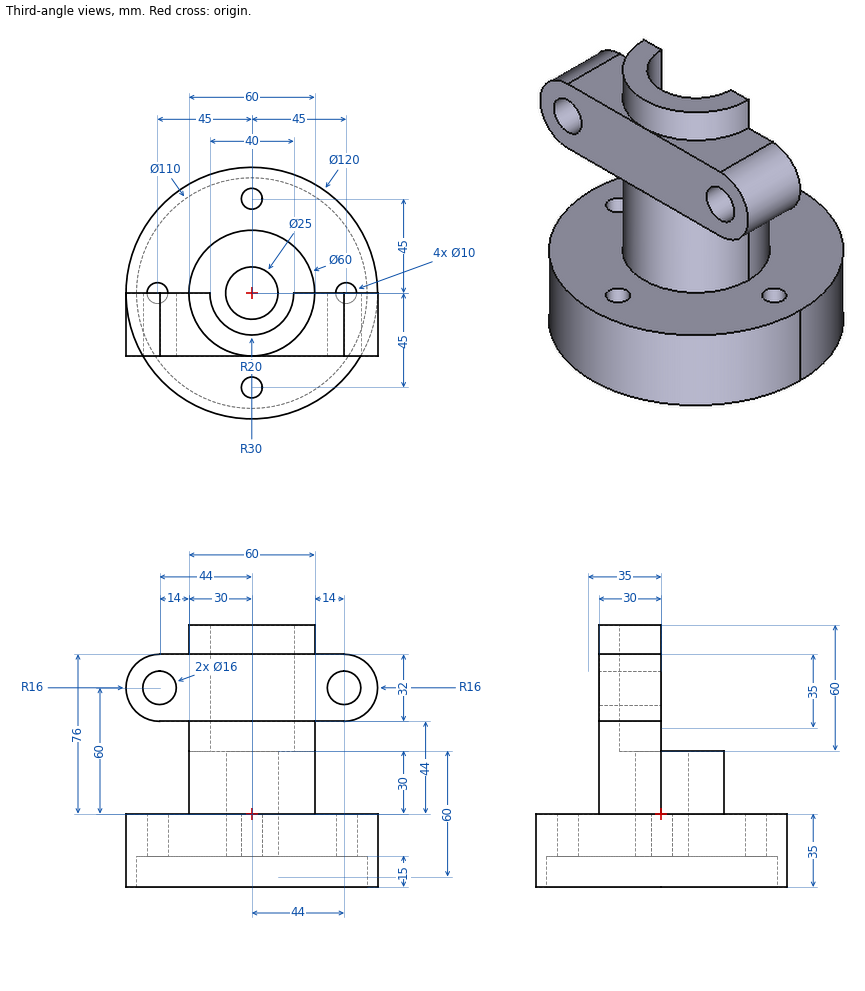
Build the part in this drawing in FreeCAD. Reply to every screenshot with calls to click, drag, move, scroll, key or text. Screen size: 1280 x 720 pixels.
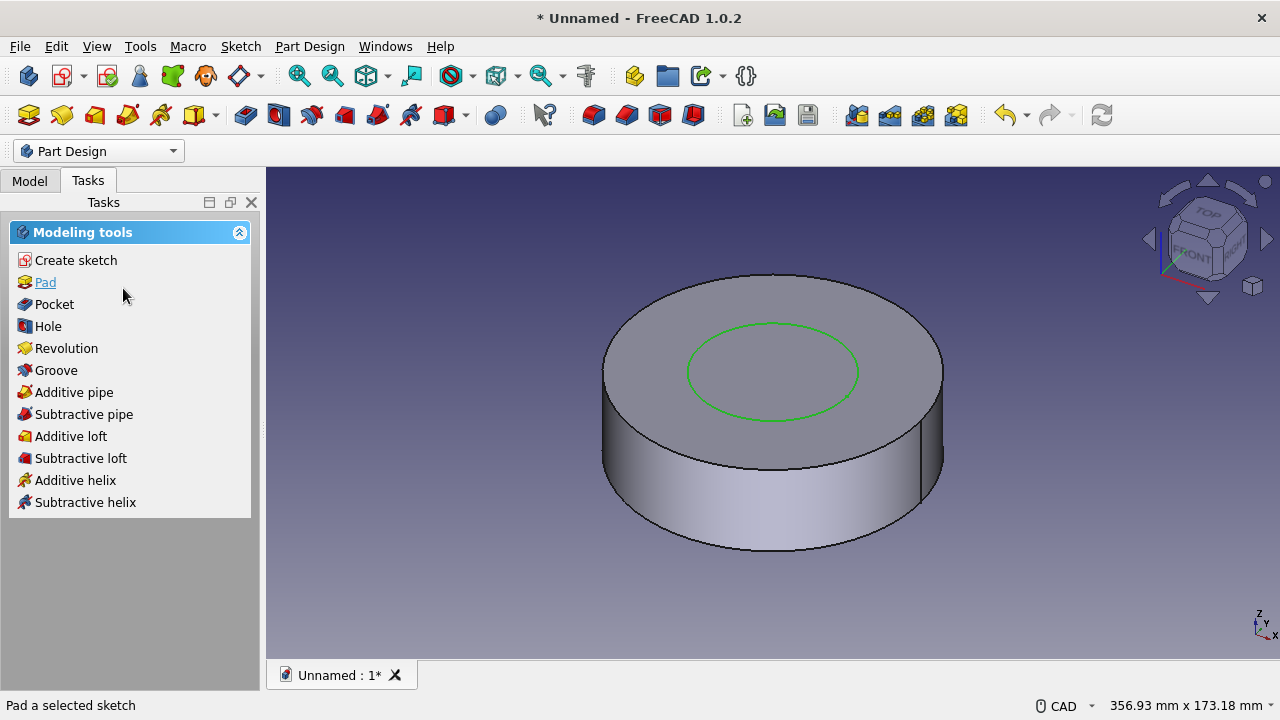
click(29, 116)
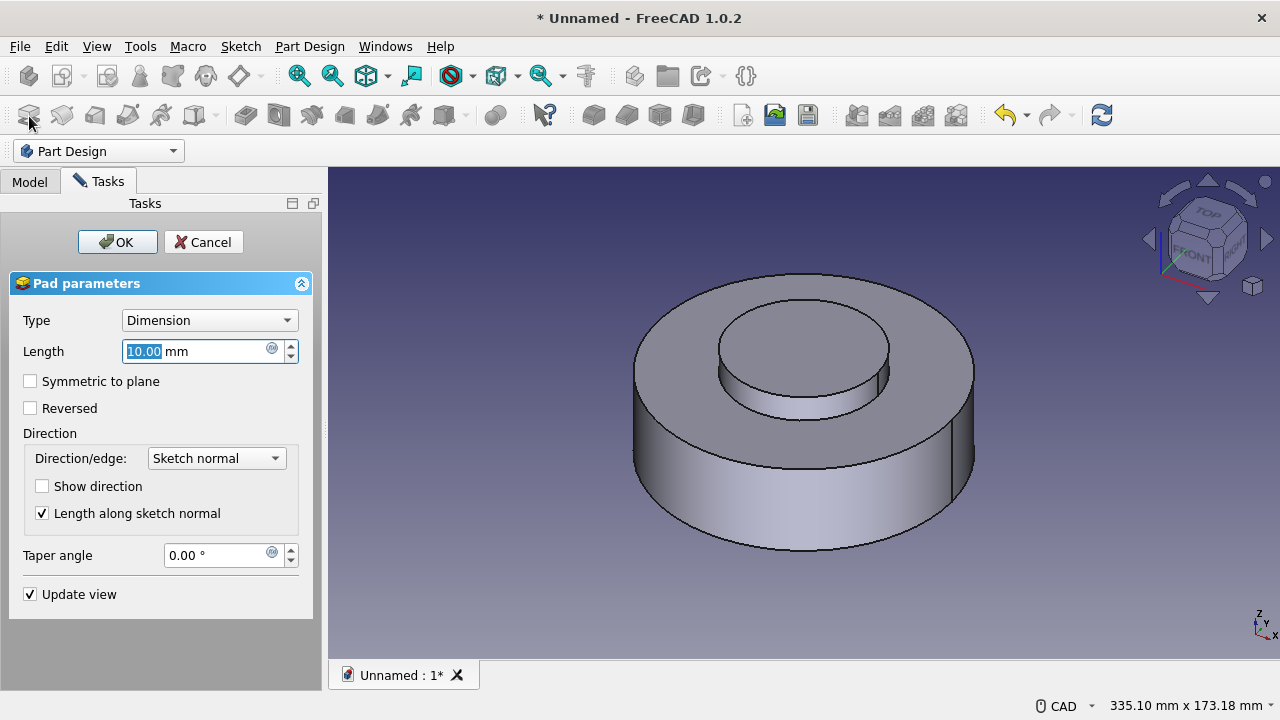
text(30)
key(Tab)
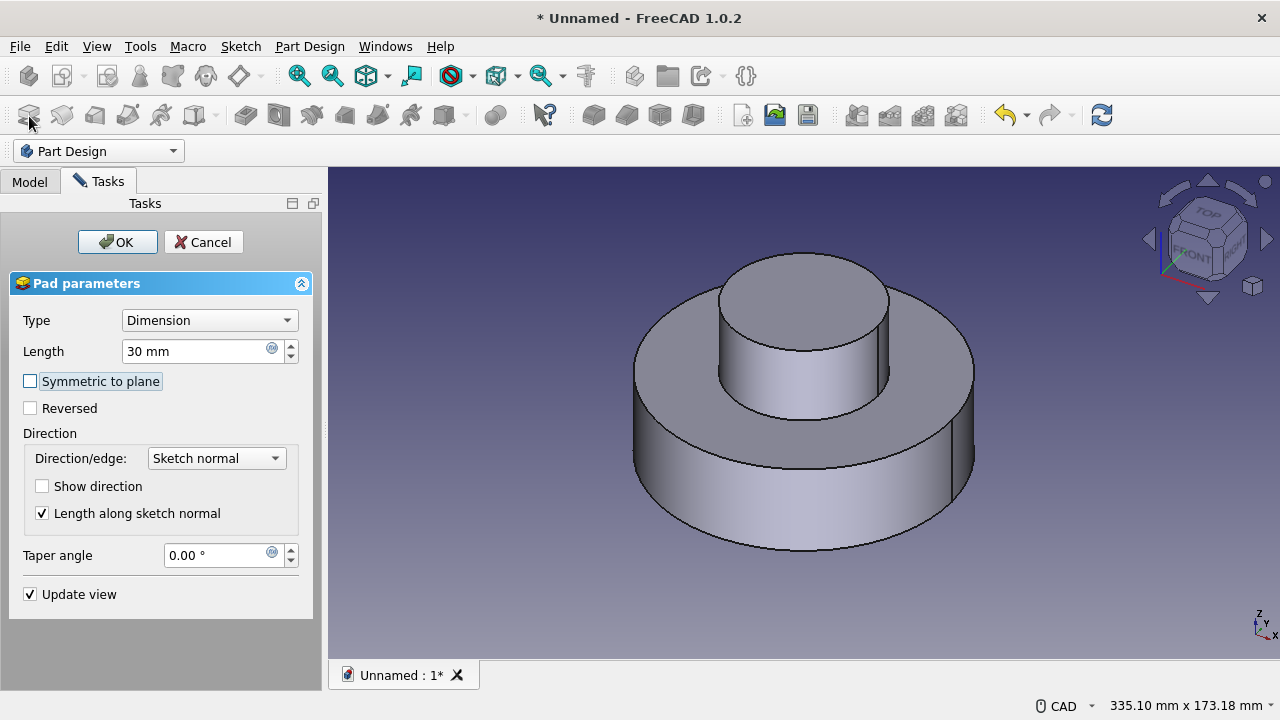
click(118, 242)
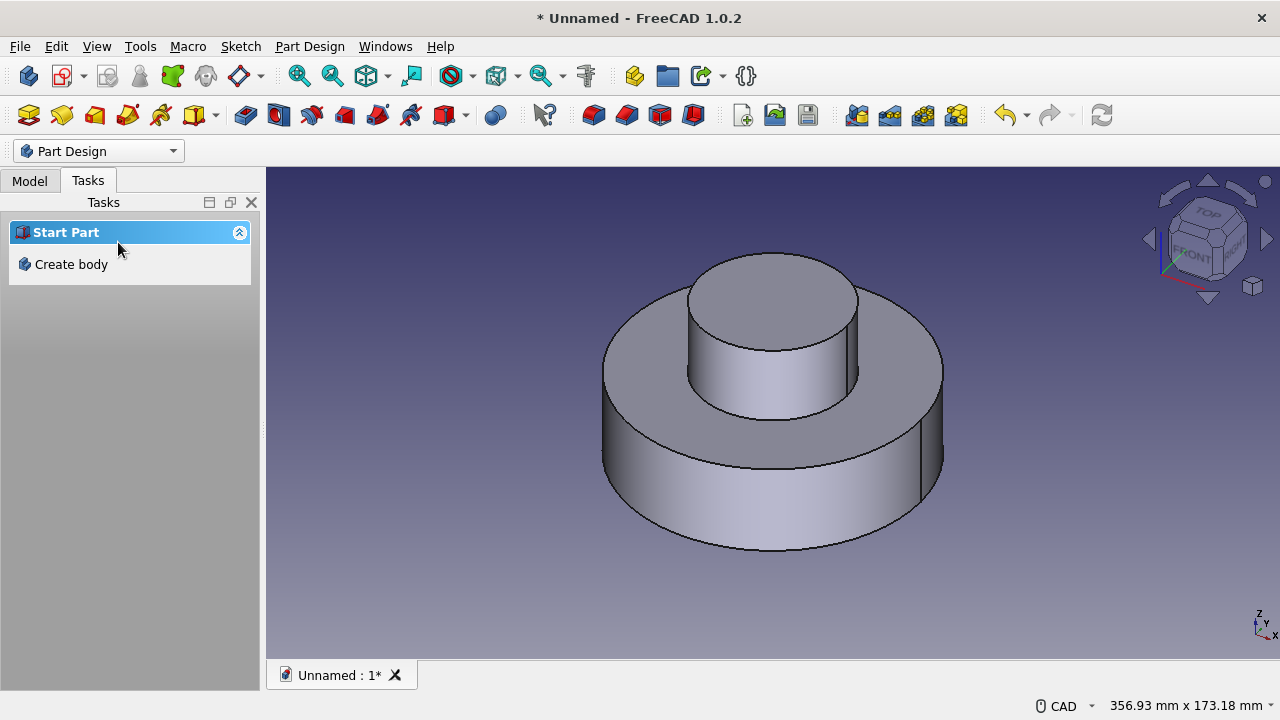
click(773, 301)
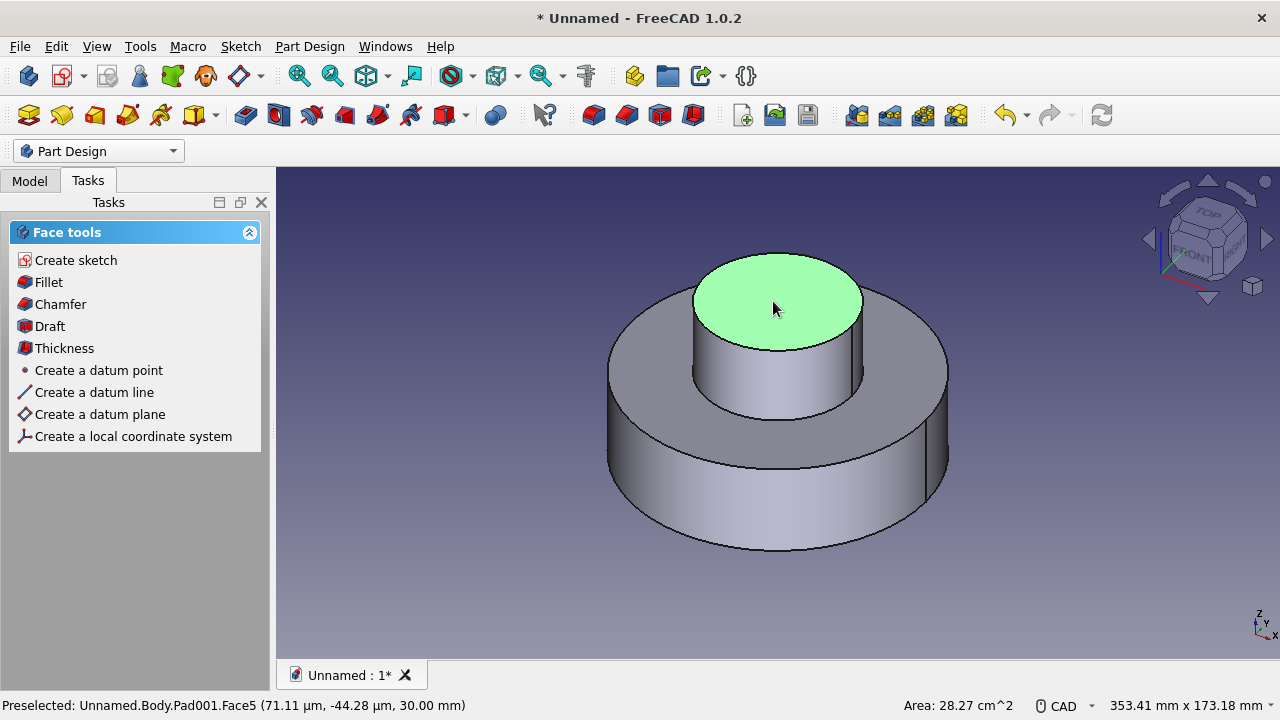
click(62, 76)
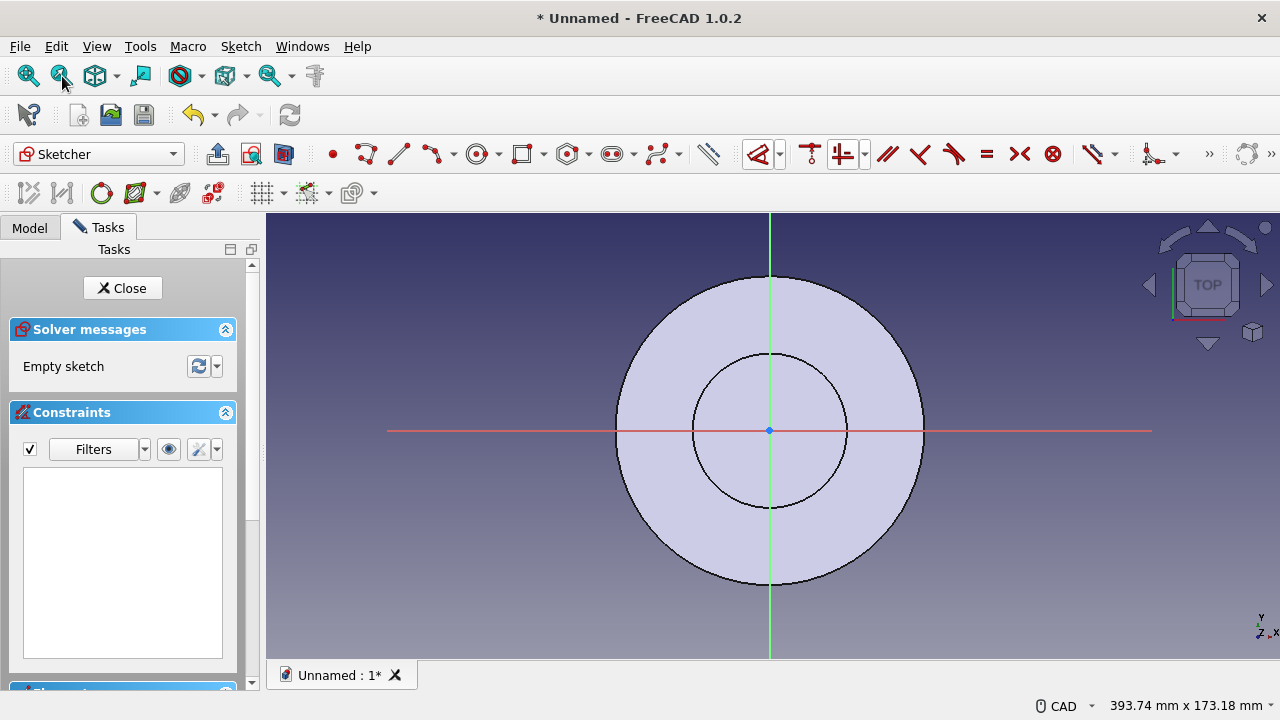
scroll(798, 484, up, 6)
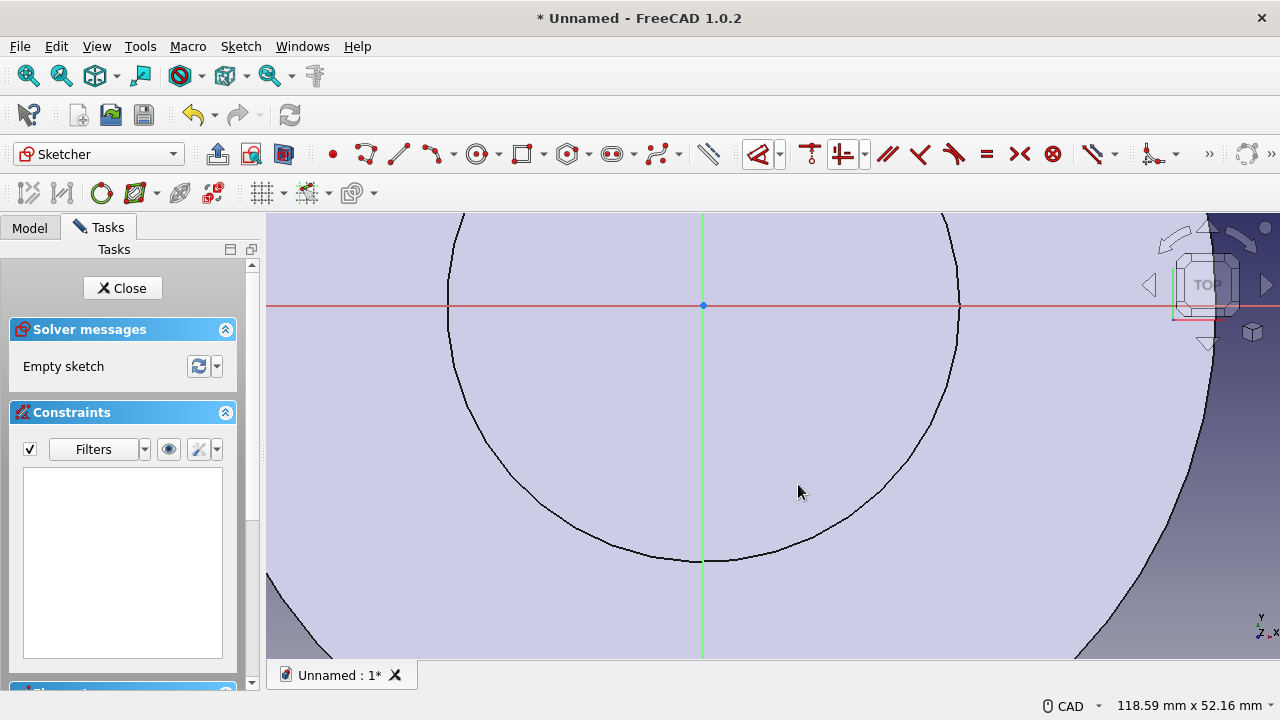
click(399, 154)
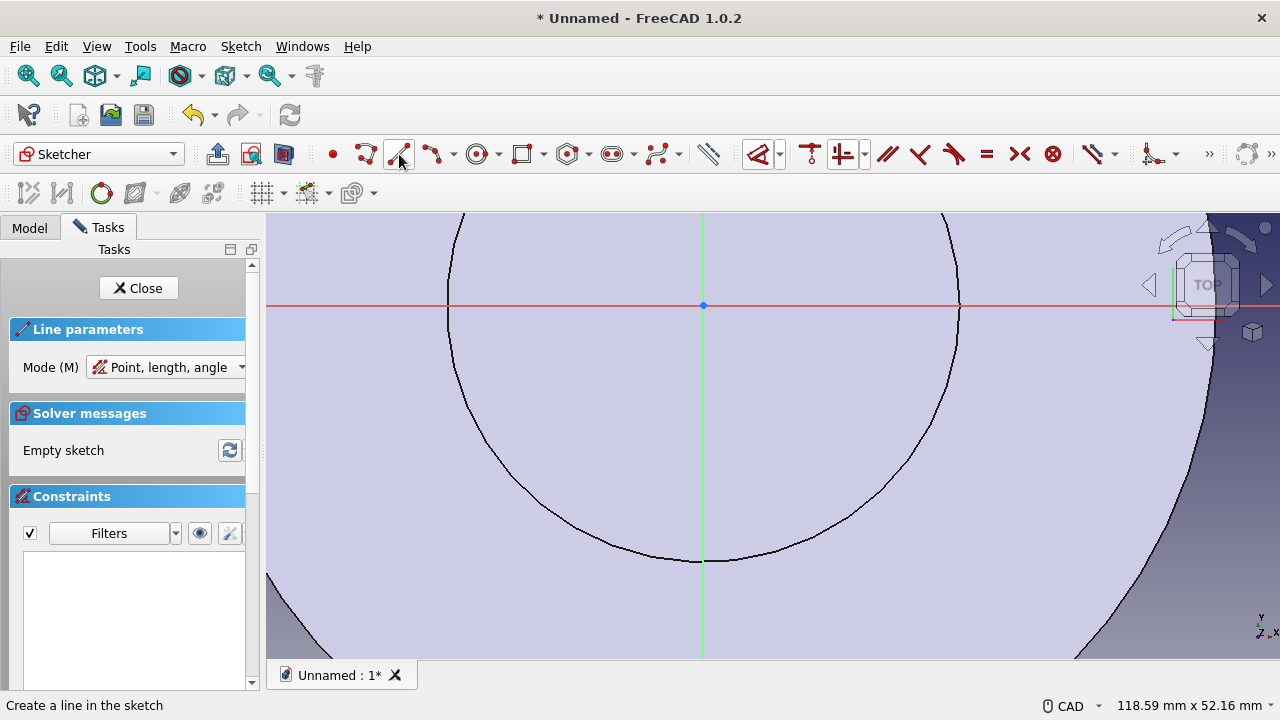
click(960, 306)
click(447, 315)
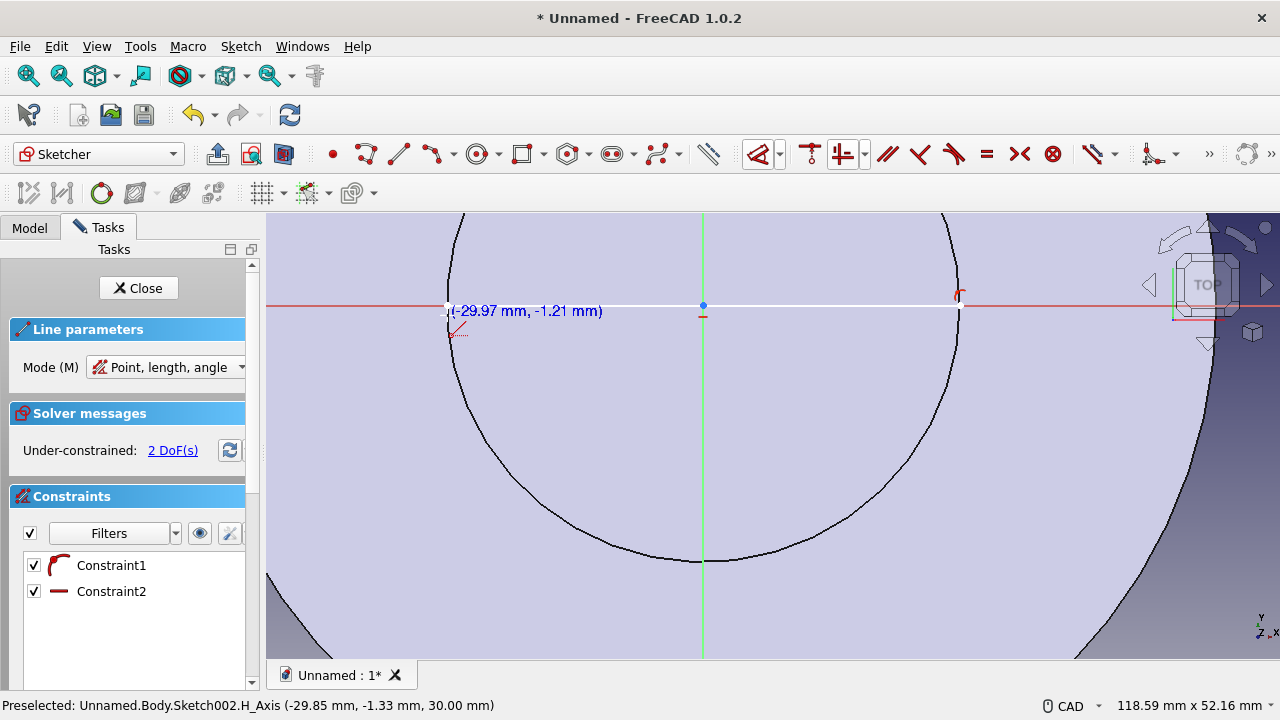
click(432, 154)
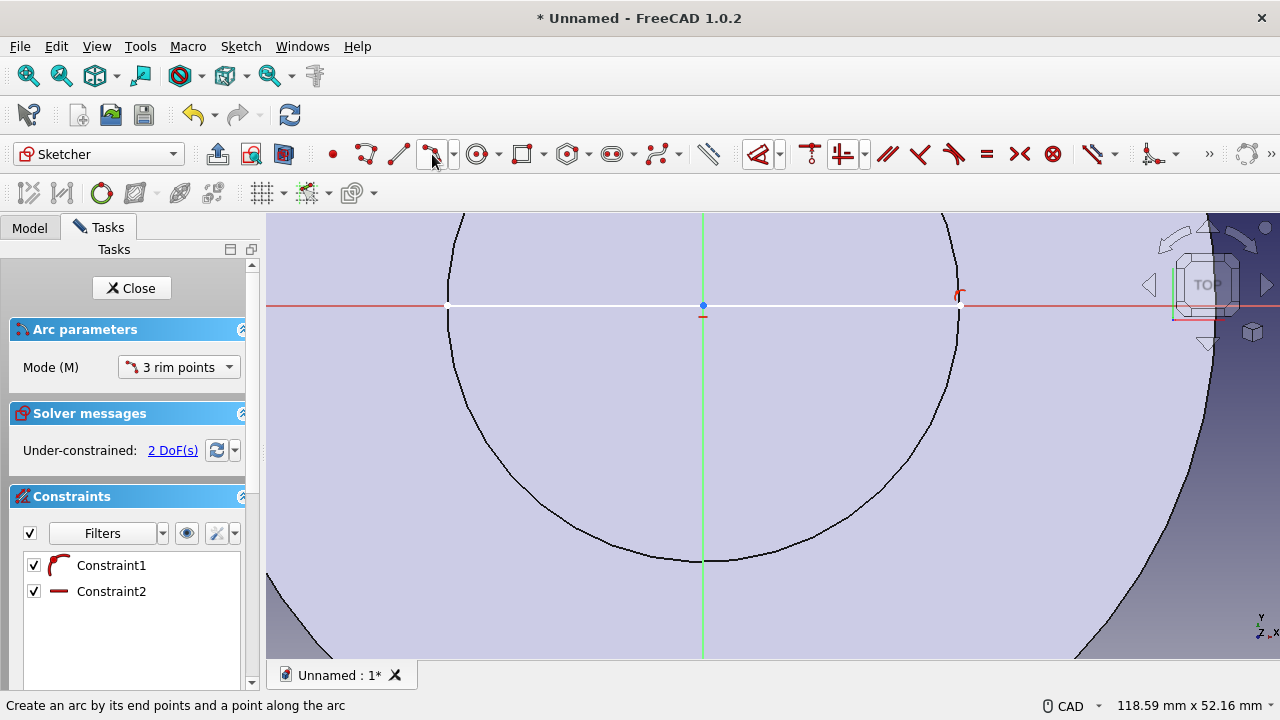
click(447, 315)
click(960, 306)
click(624, 550)
key(Escape)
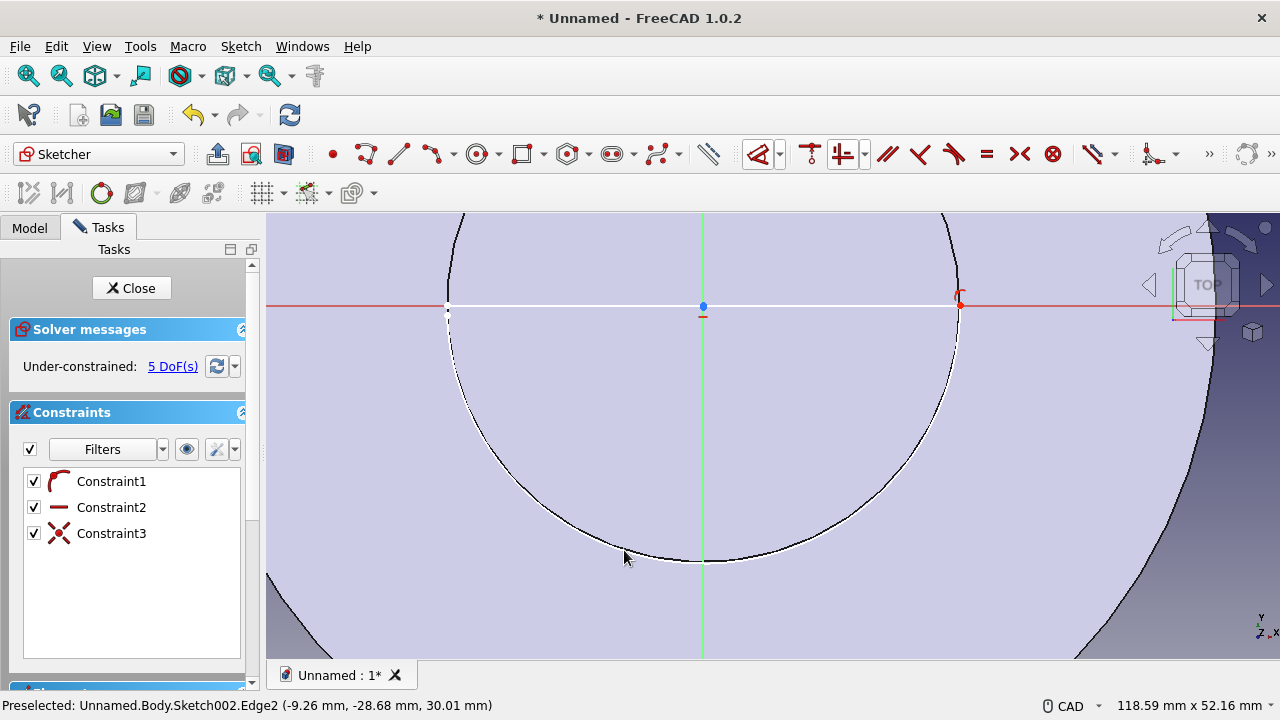
drag(693, 296, 713, 317)